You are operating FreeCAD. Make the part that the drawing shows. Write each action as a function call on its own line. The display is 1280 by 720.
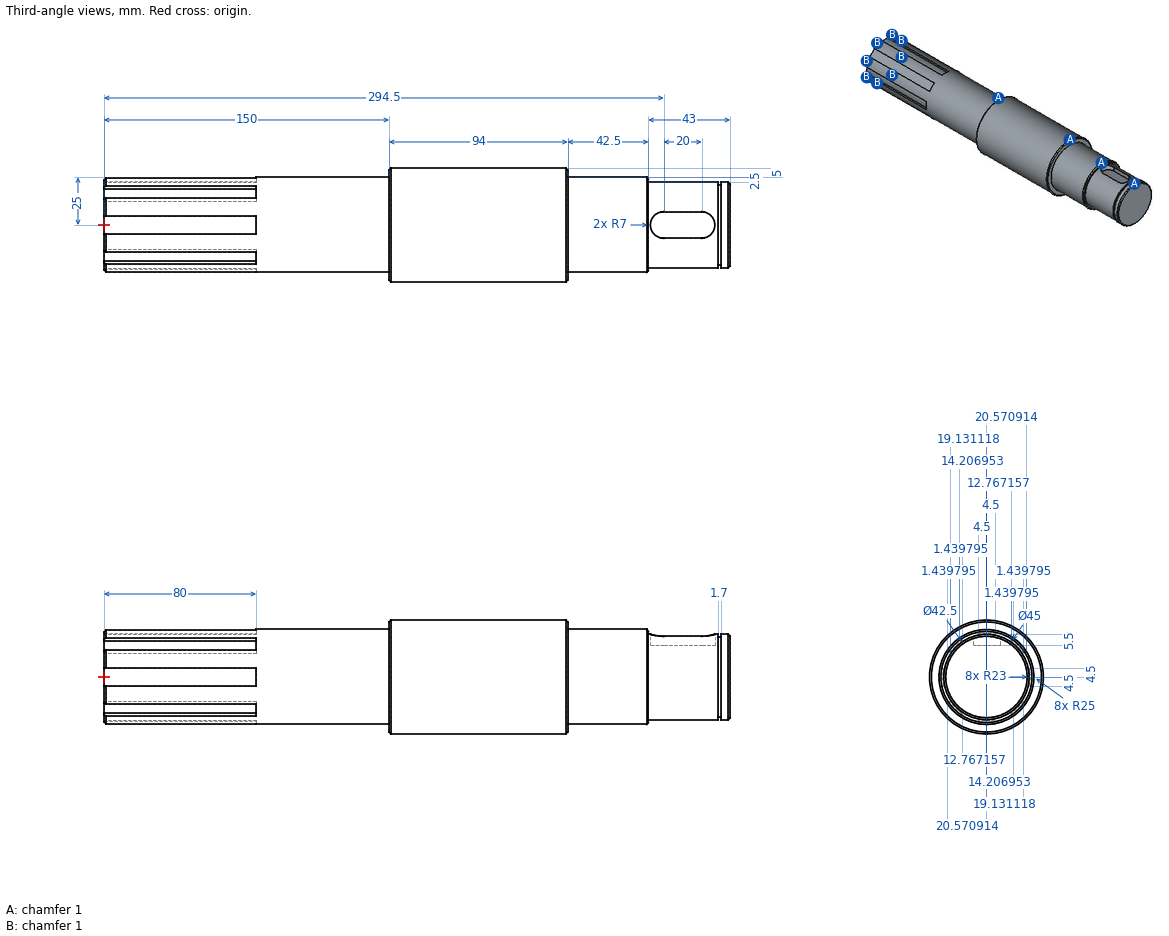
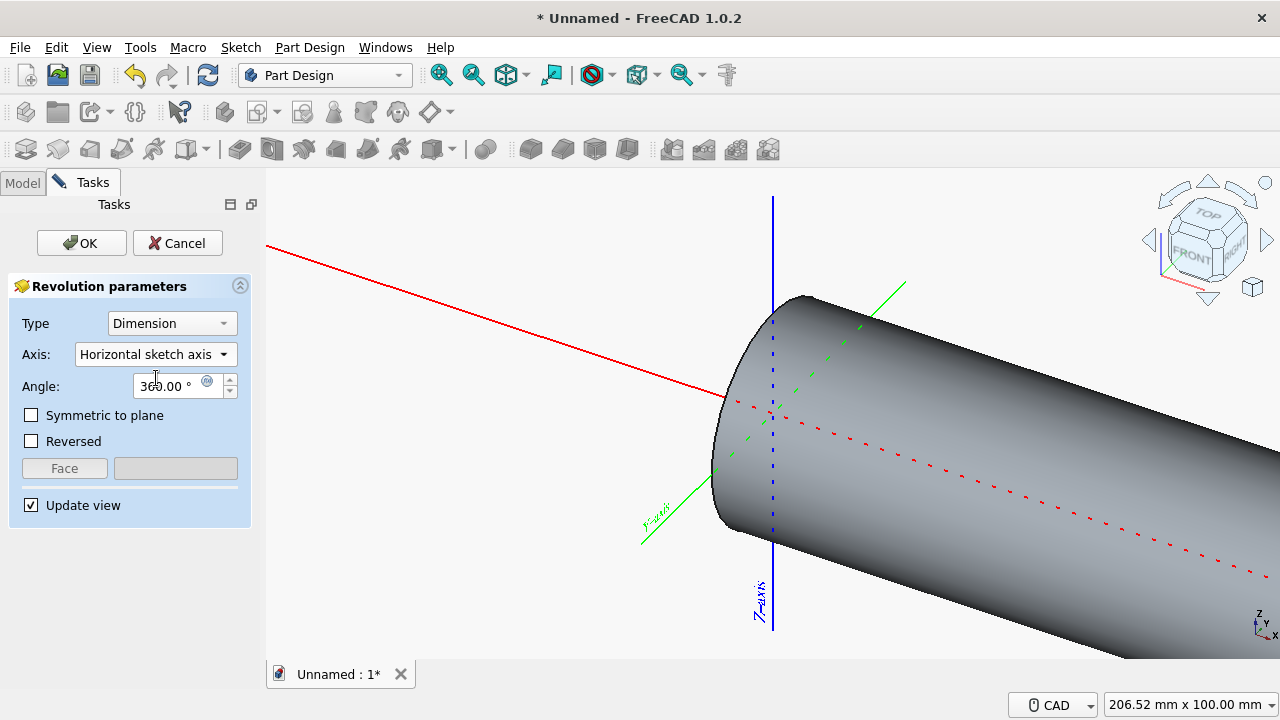
click(82, 243)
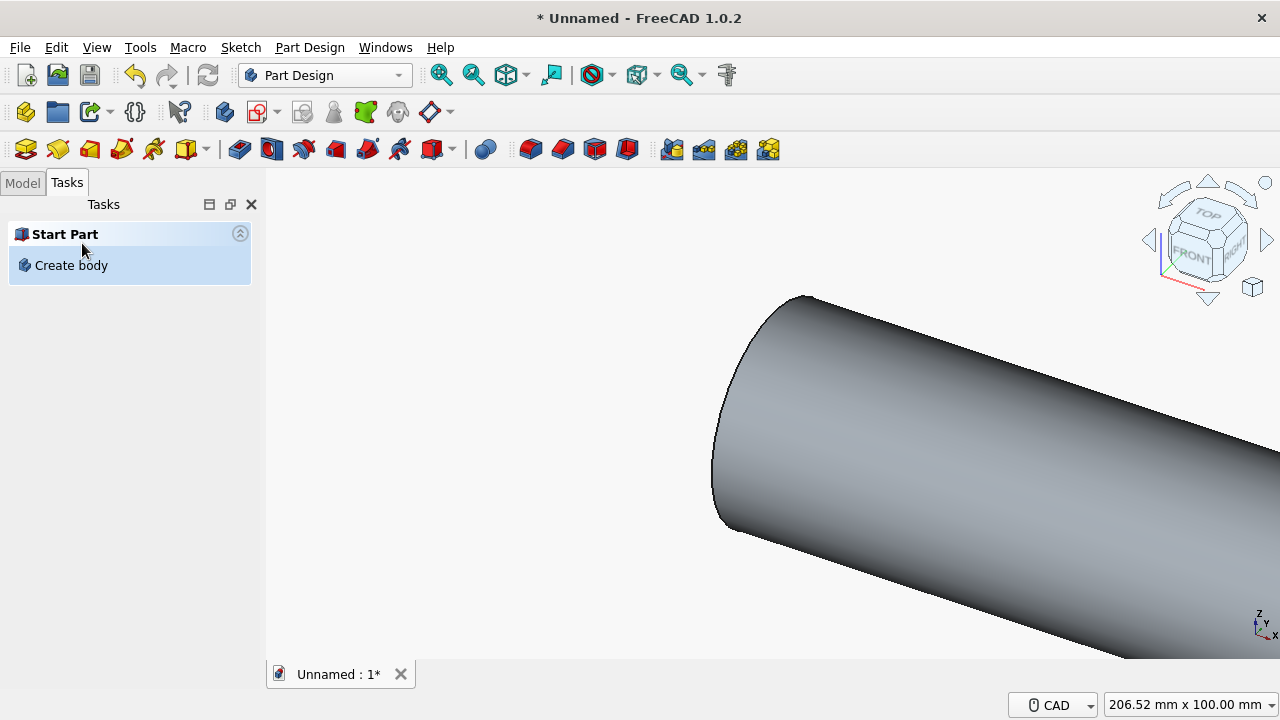
click(442, 76)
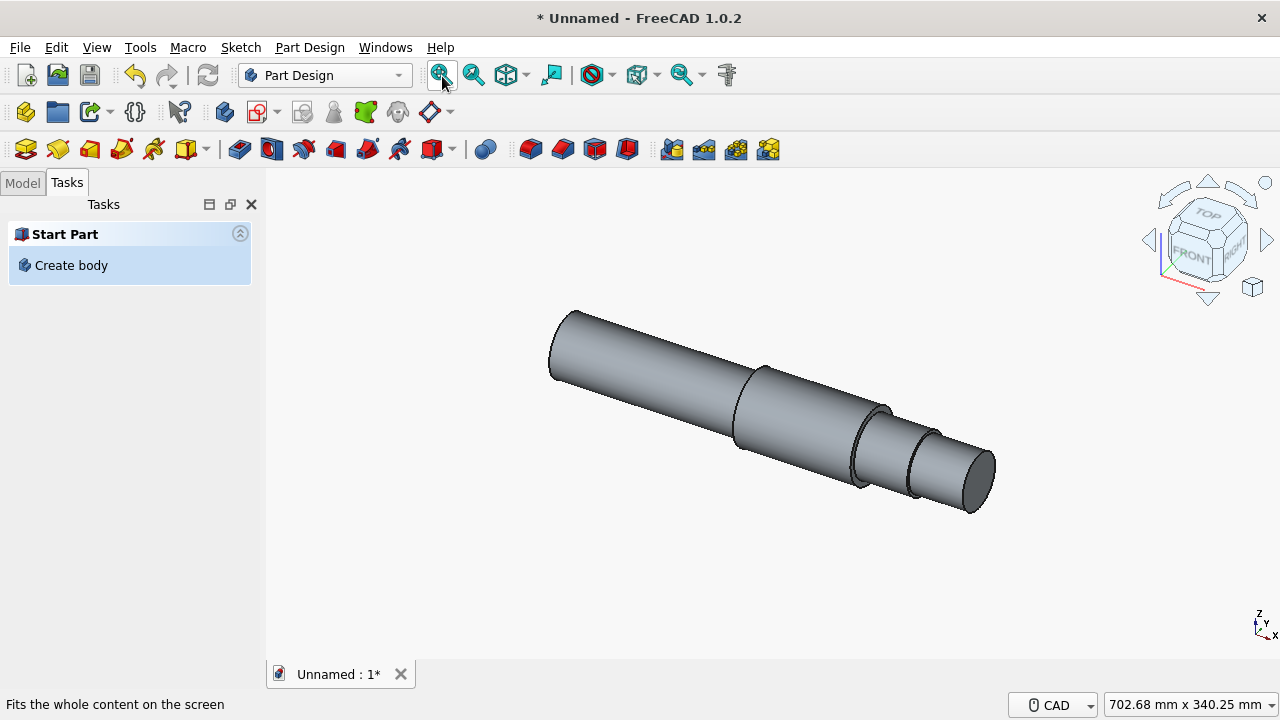
click(963, 497)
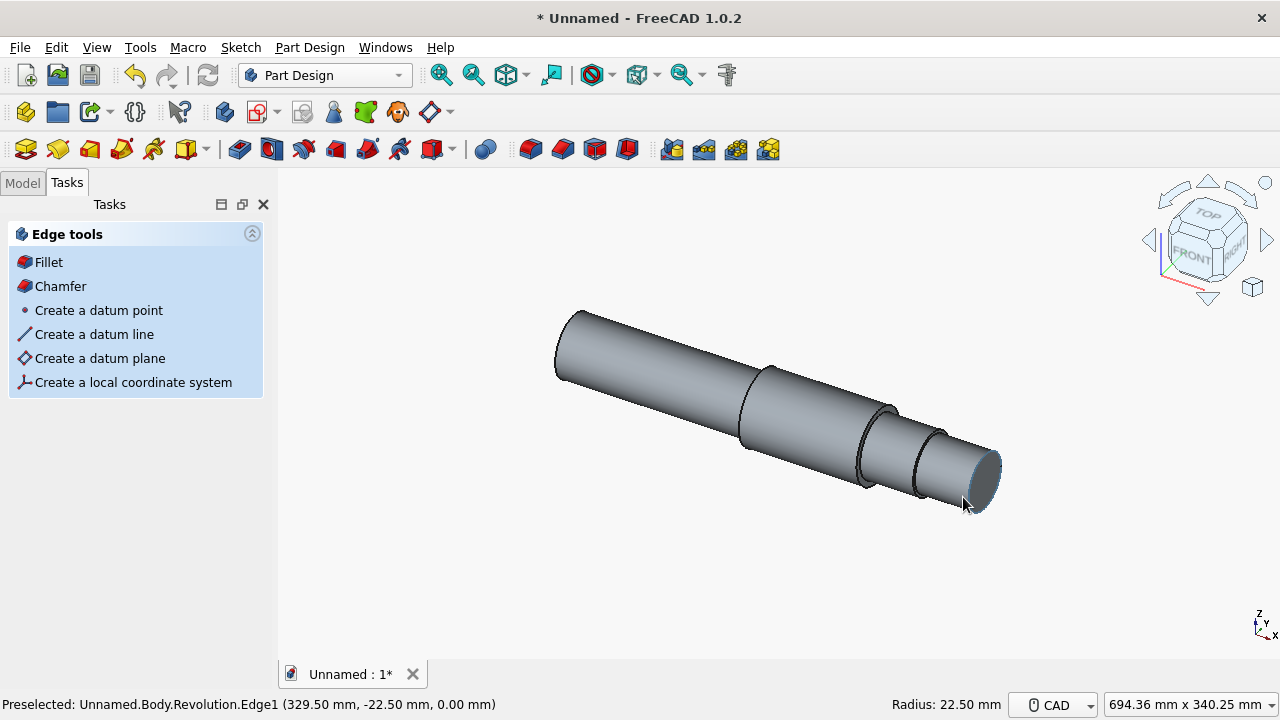
click(913, 481, ctrl)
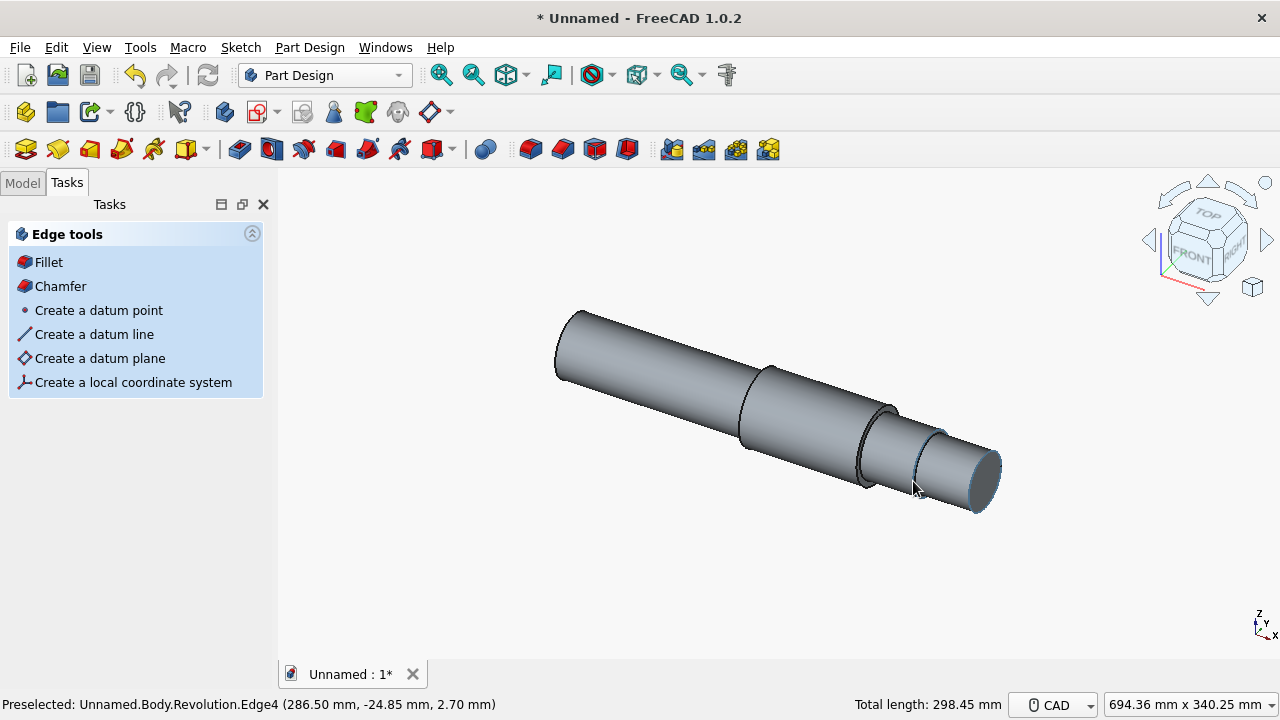
click(856, 467, ctrl)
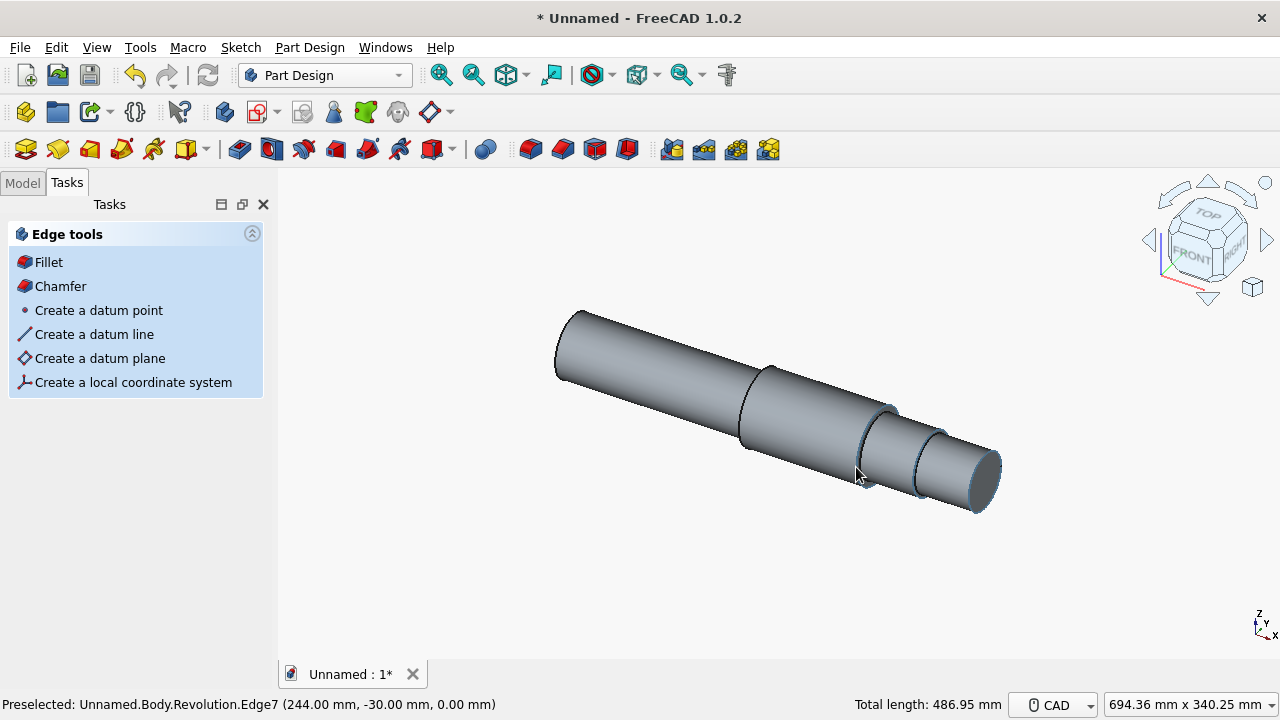
click(767, 366, ctrl)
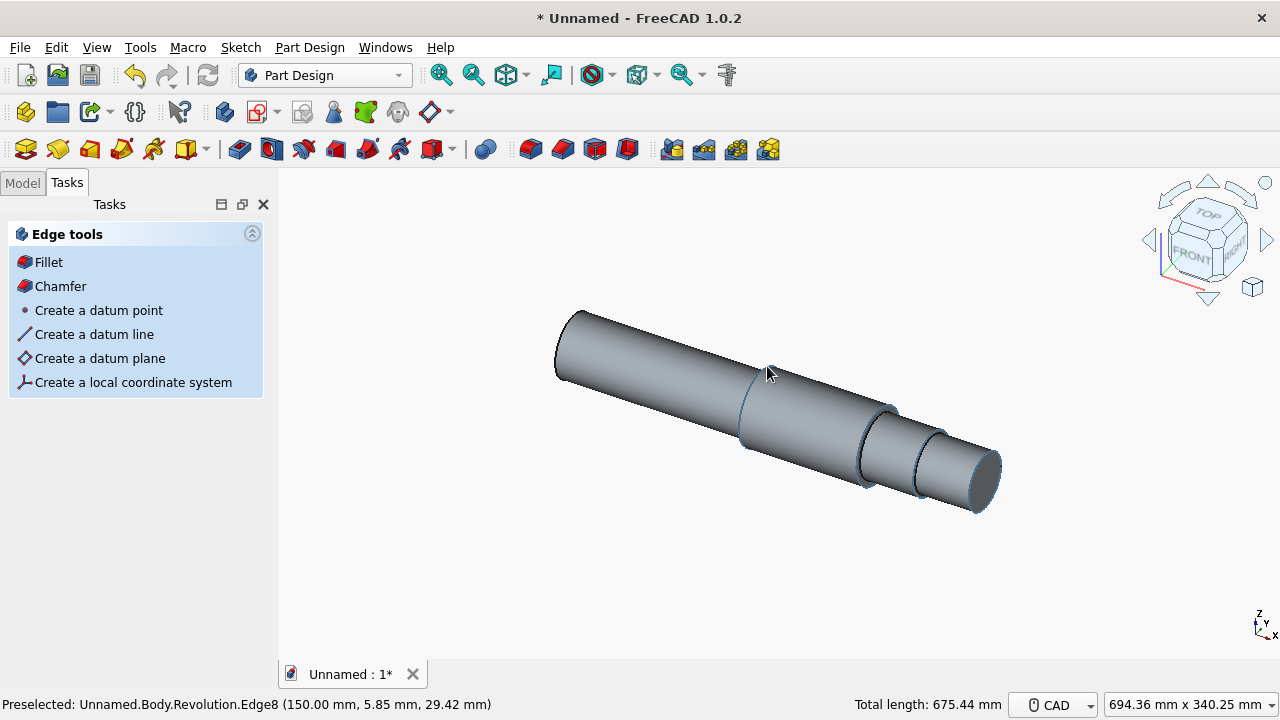
click(564, 150)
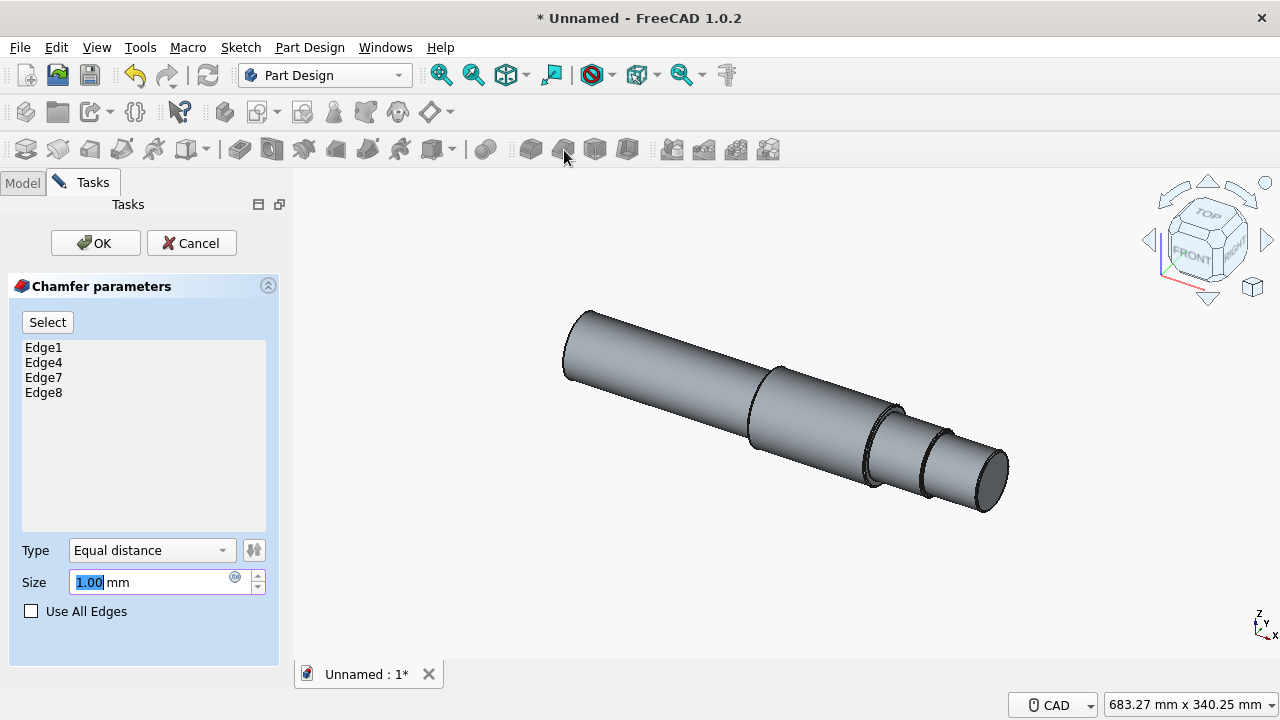
text(1)
key(Tab)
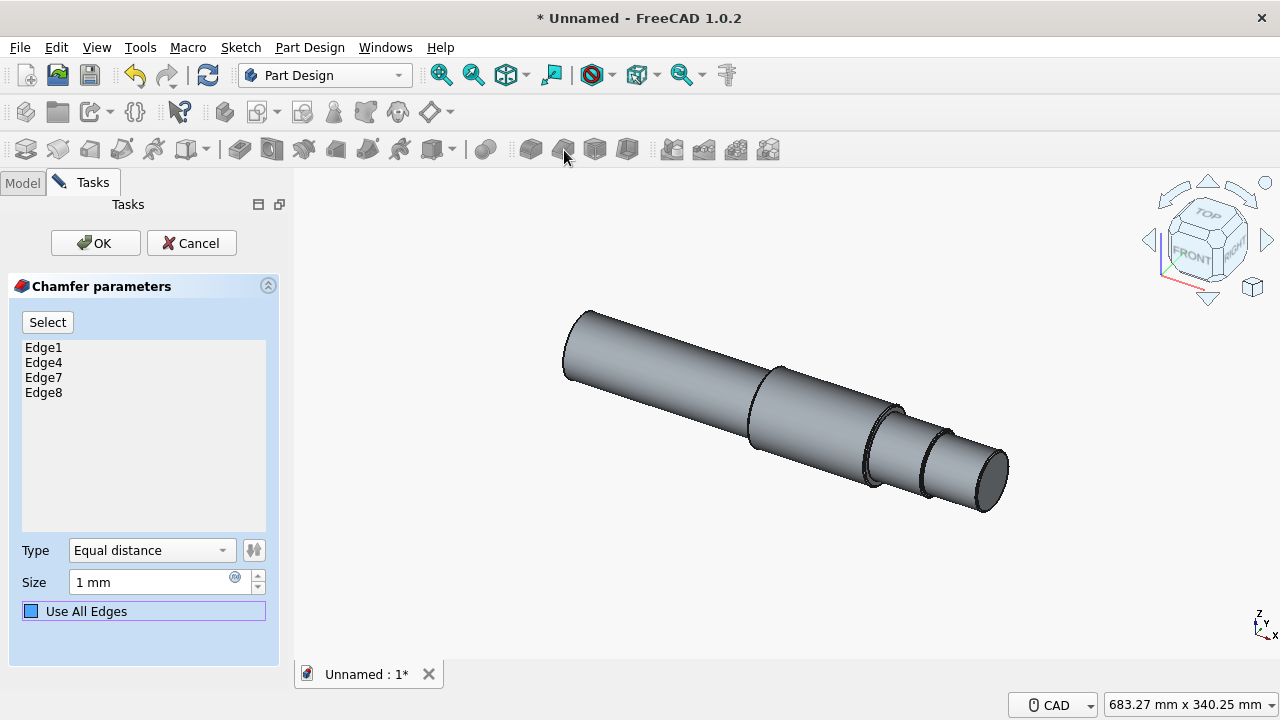
click(96, 243)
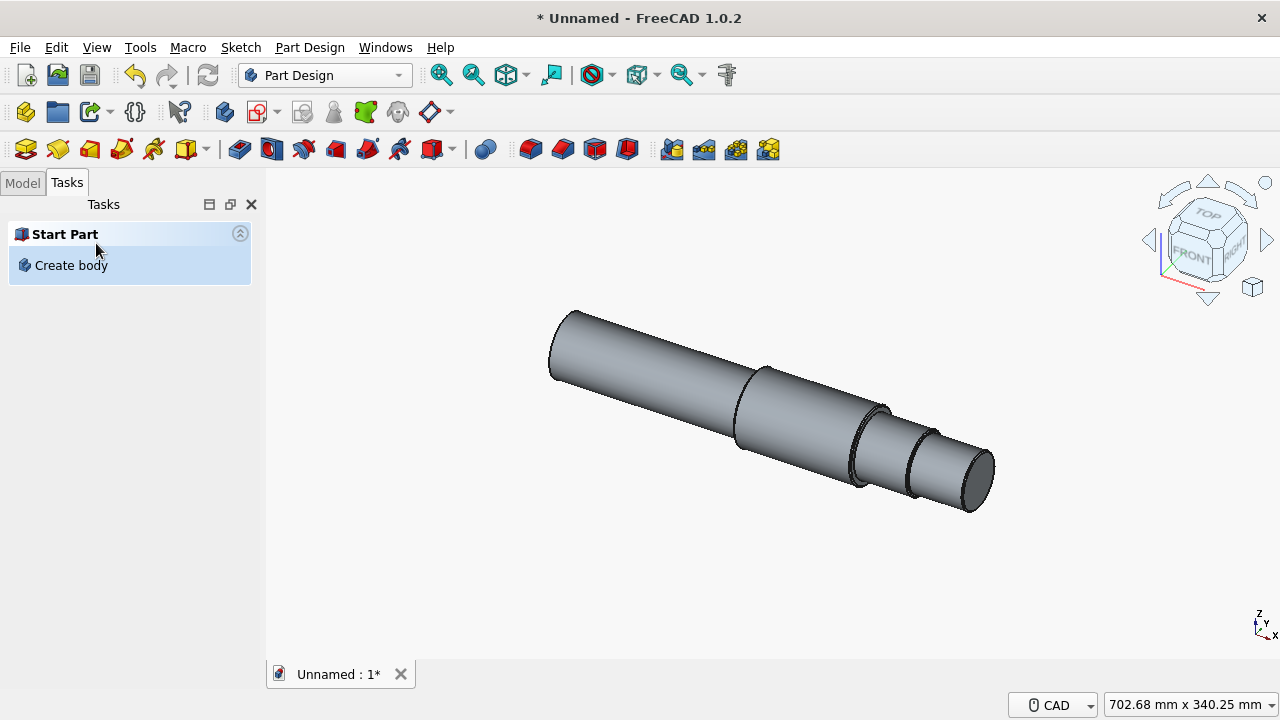
click(23, 182)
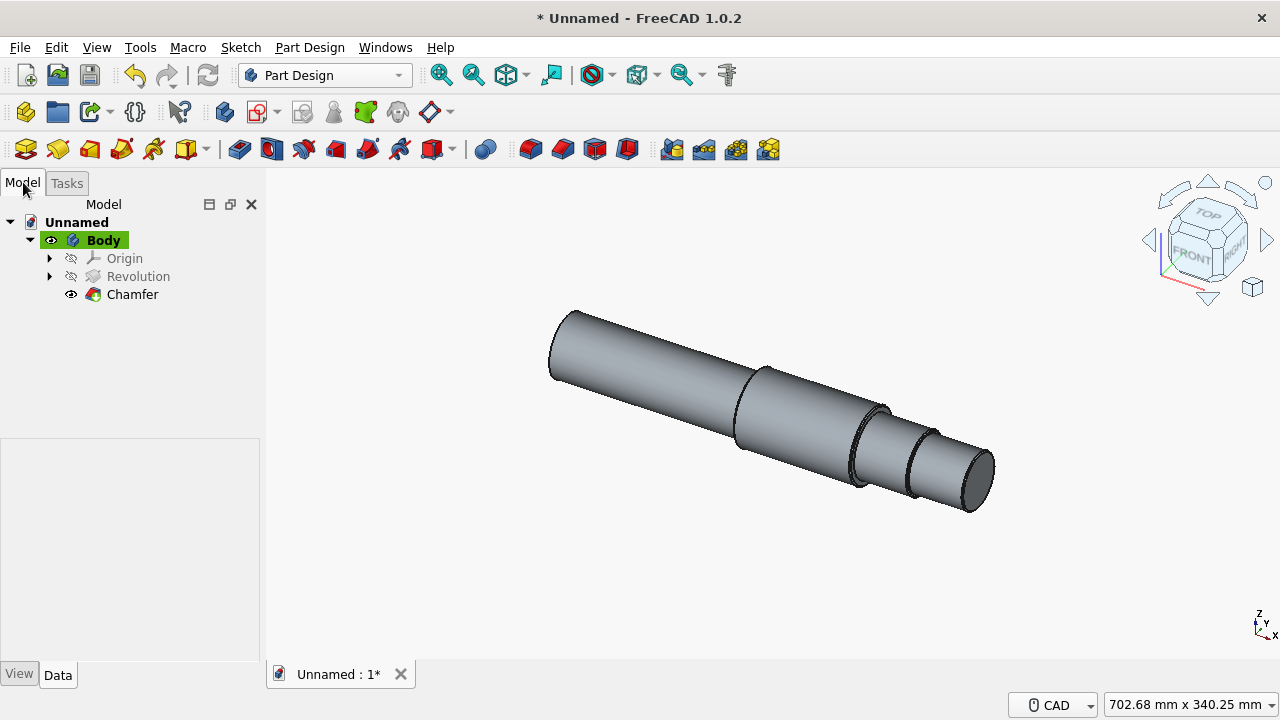
click(50, 258)